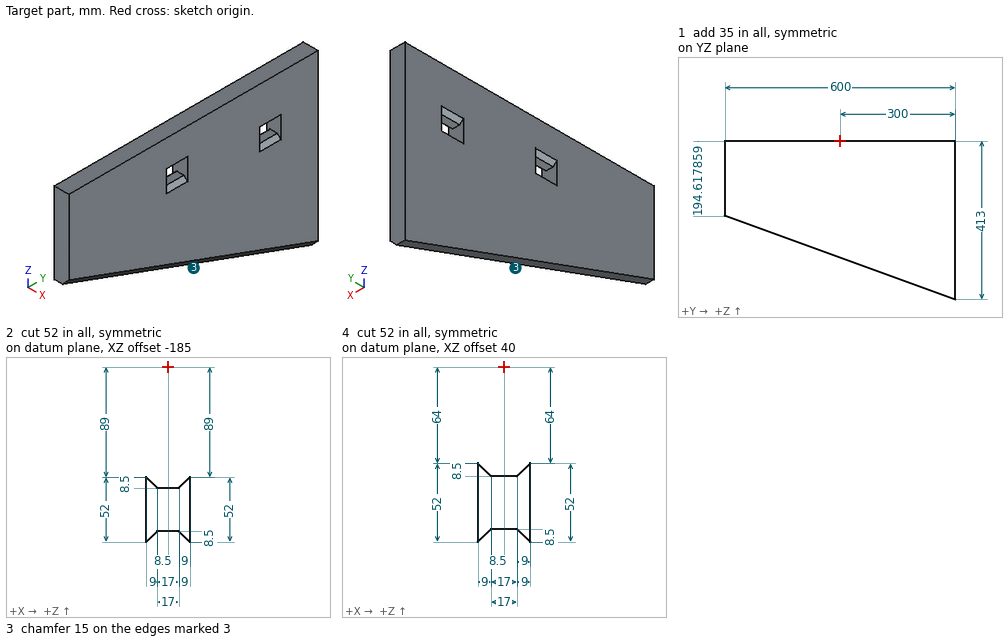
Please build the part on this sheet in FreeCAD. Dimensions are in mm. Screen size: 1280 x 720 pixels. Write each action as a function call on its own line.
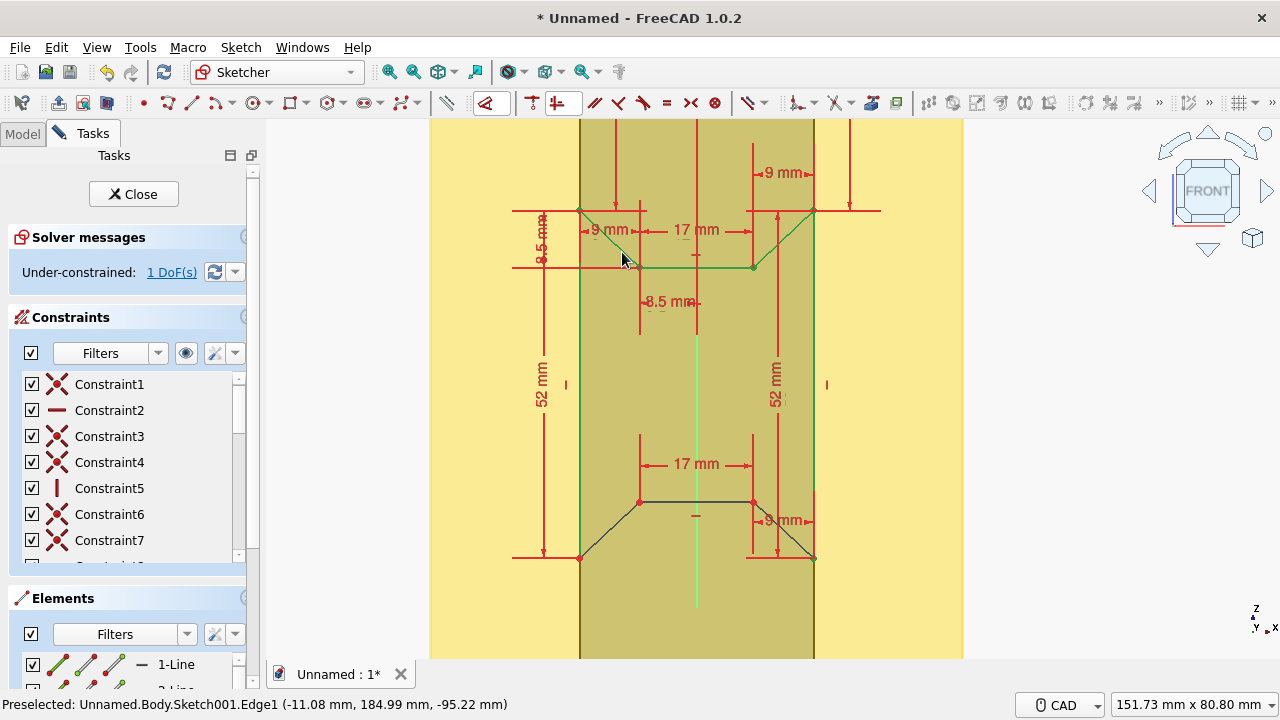
click(796, 541)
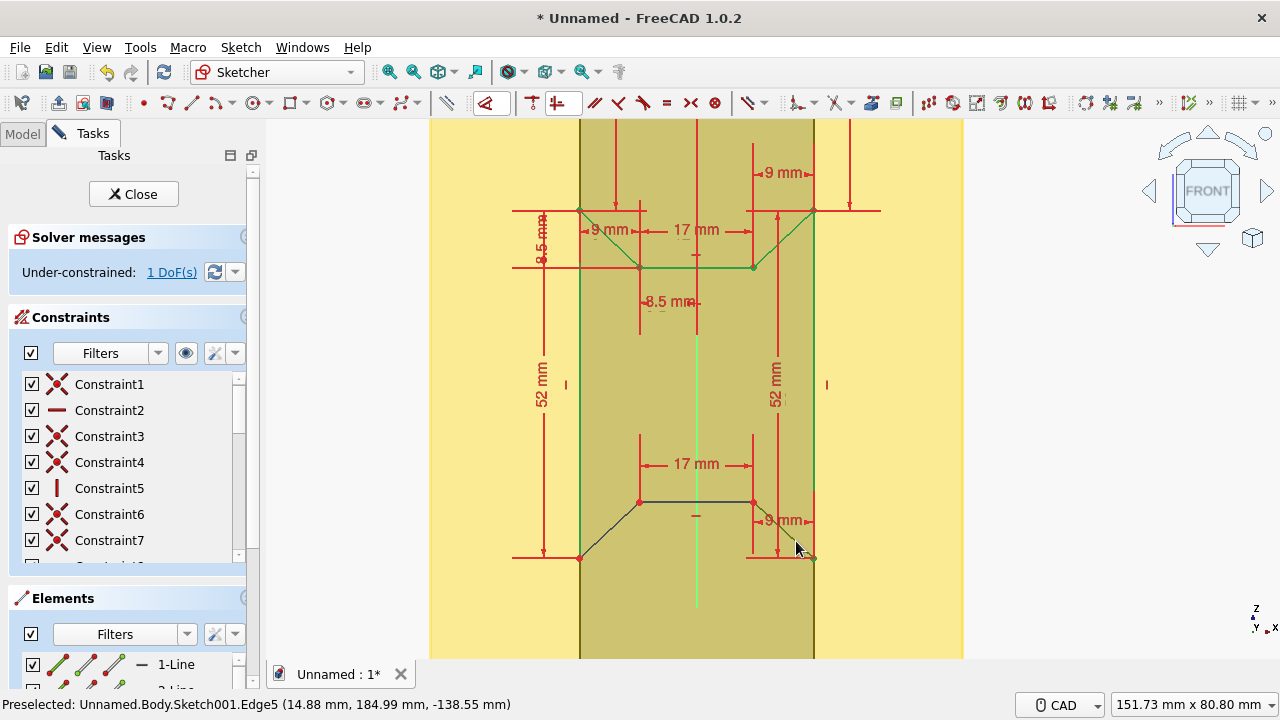
click(504, 104)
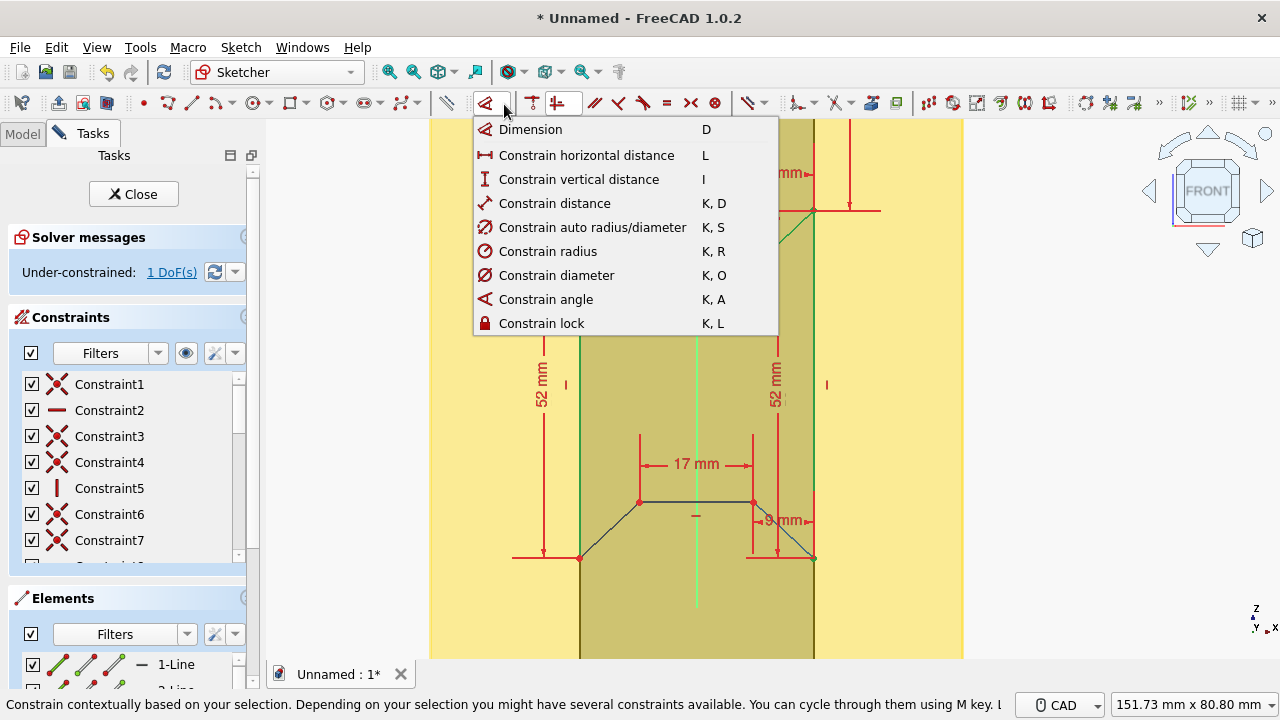
click(626, 179)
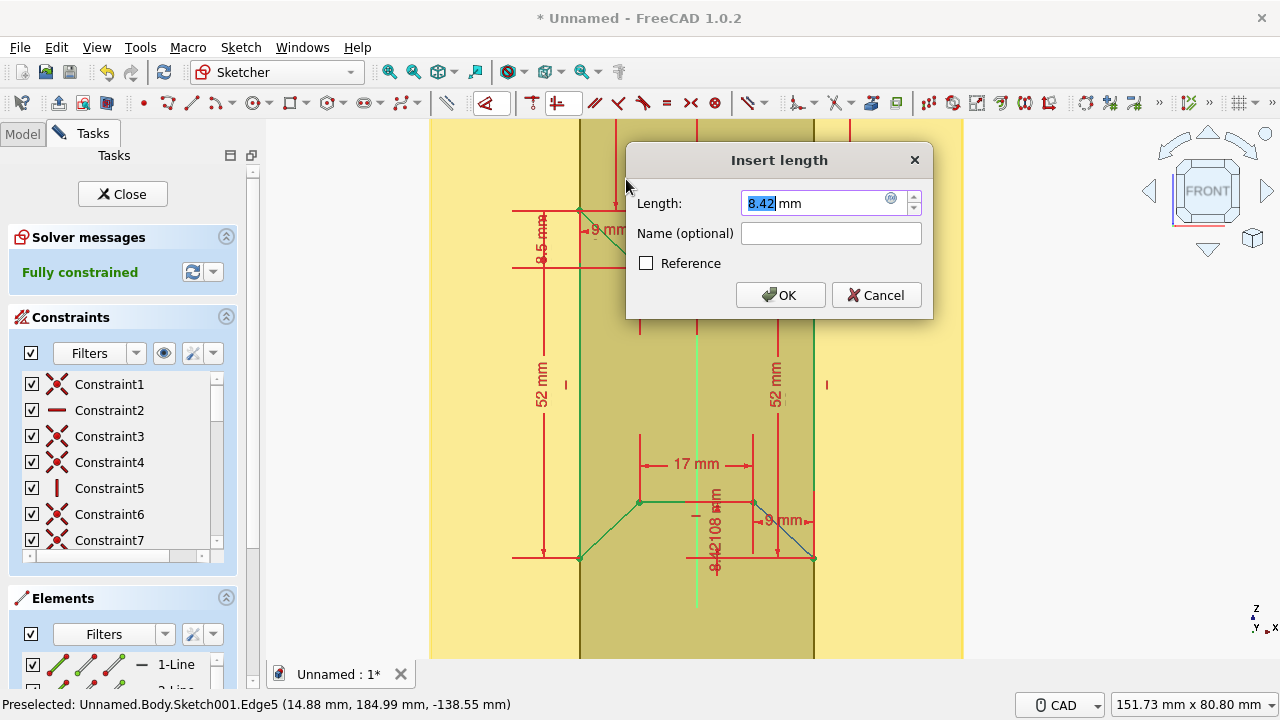
text(8.5)
key(Return)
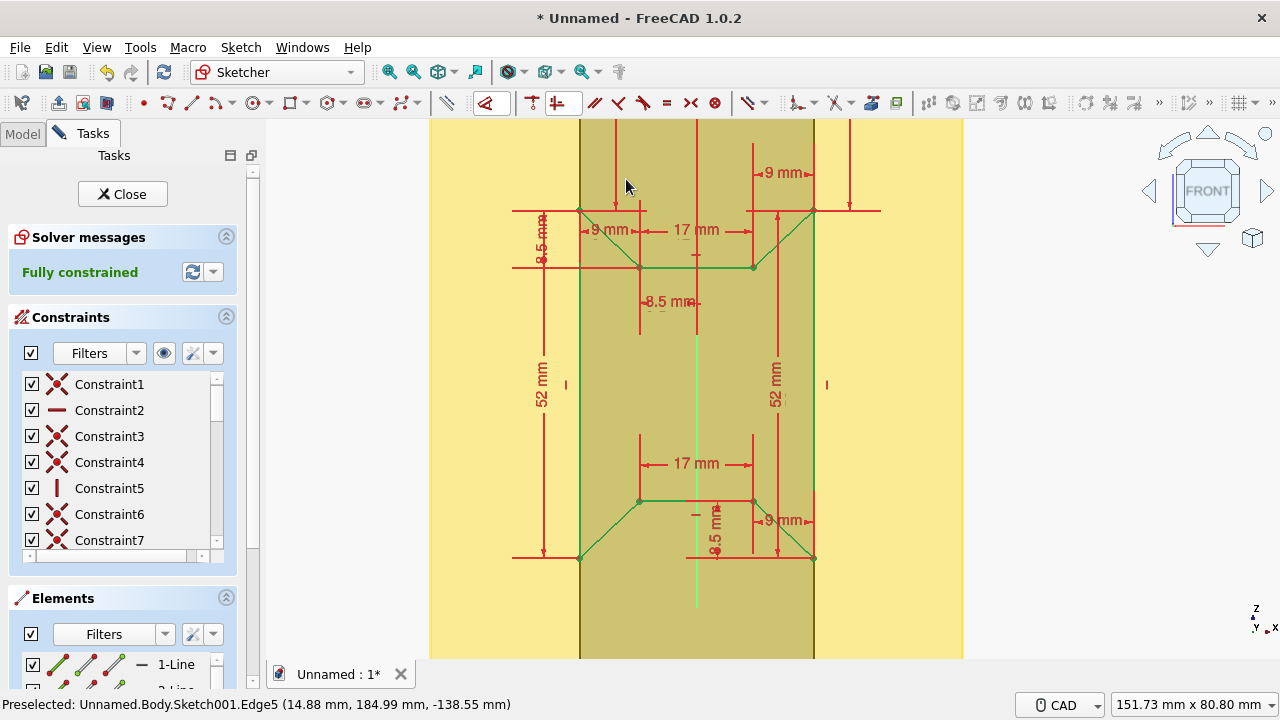
click(123, 194)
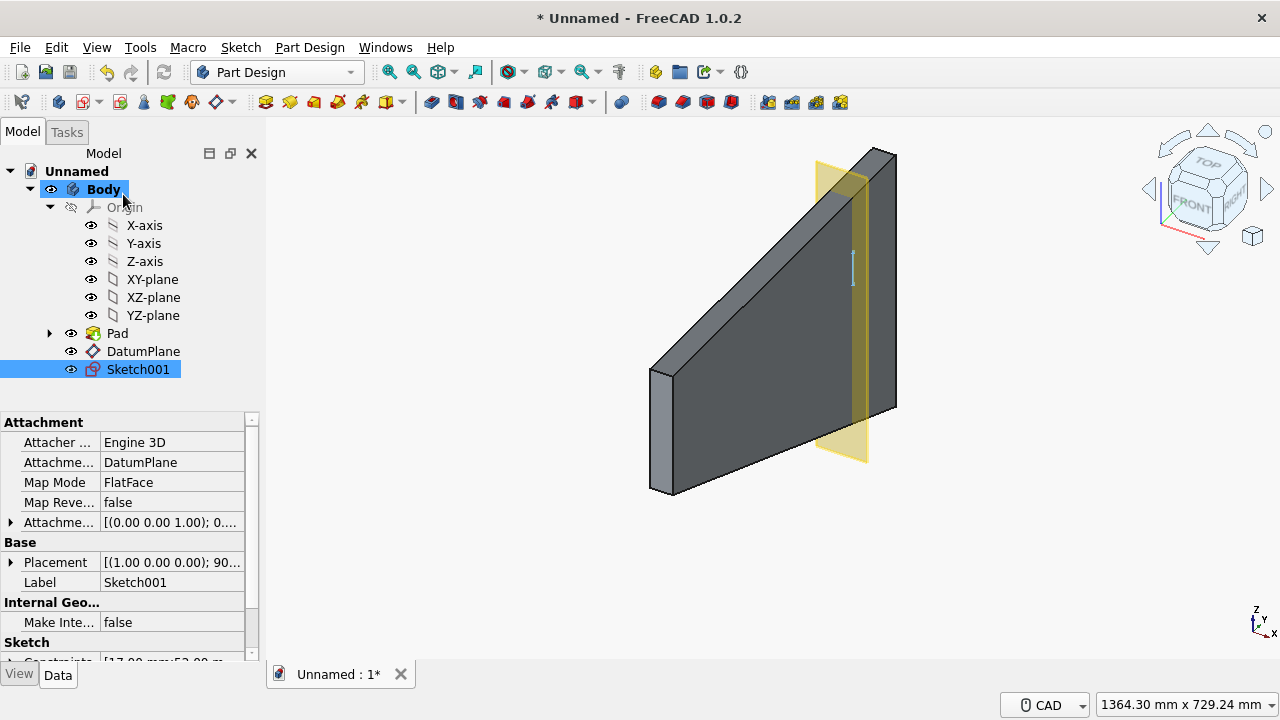
click(432, 102)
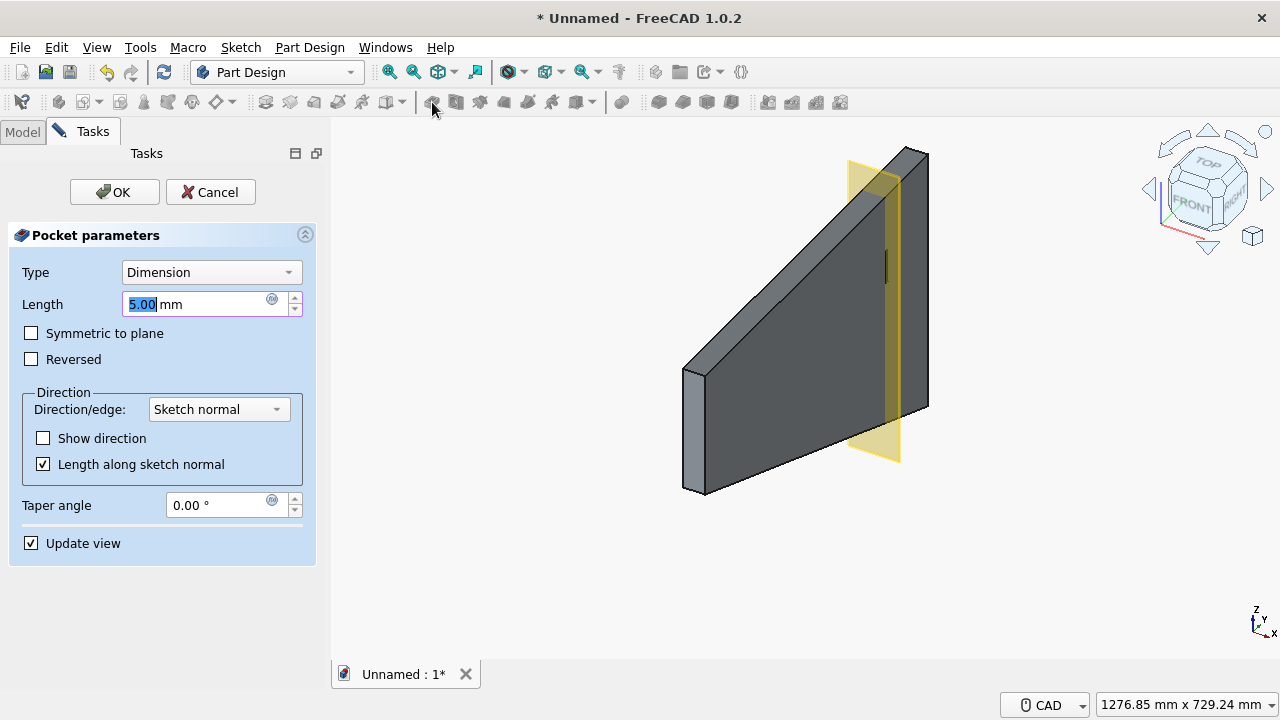
text(52)
key(Tab)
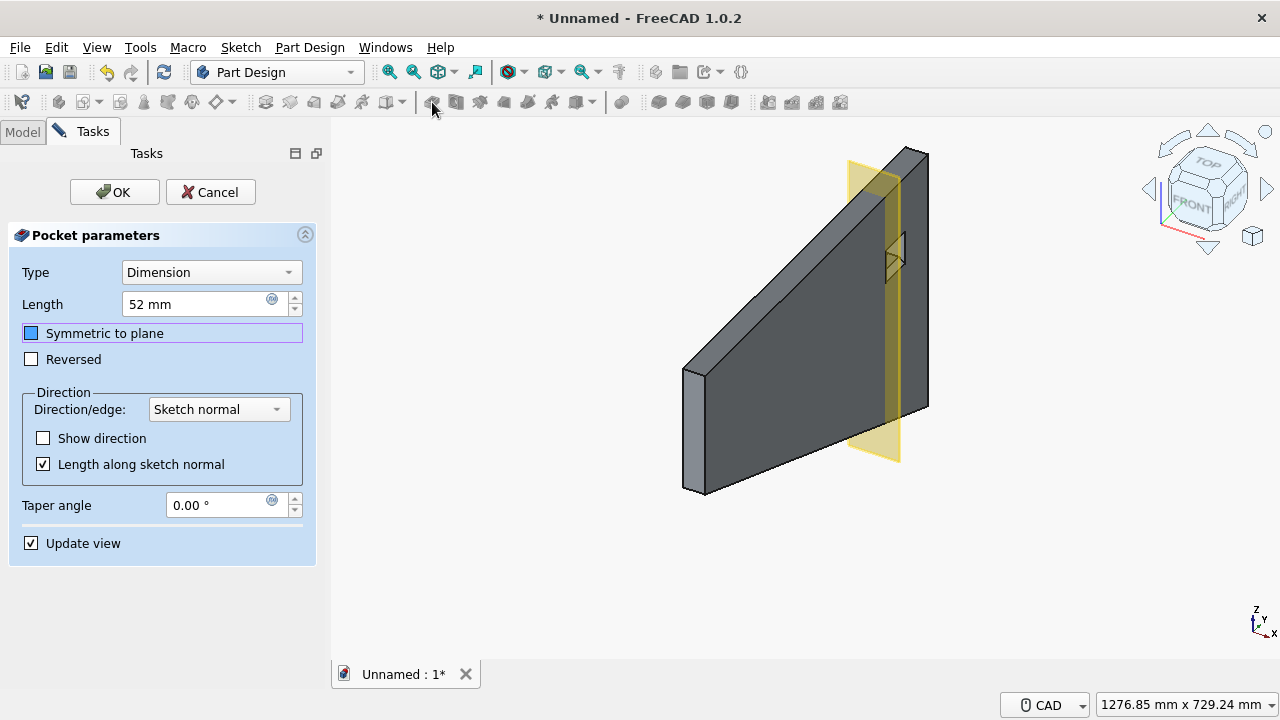
click(30, 333)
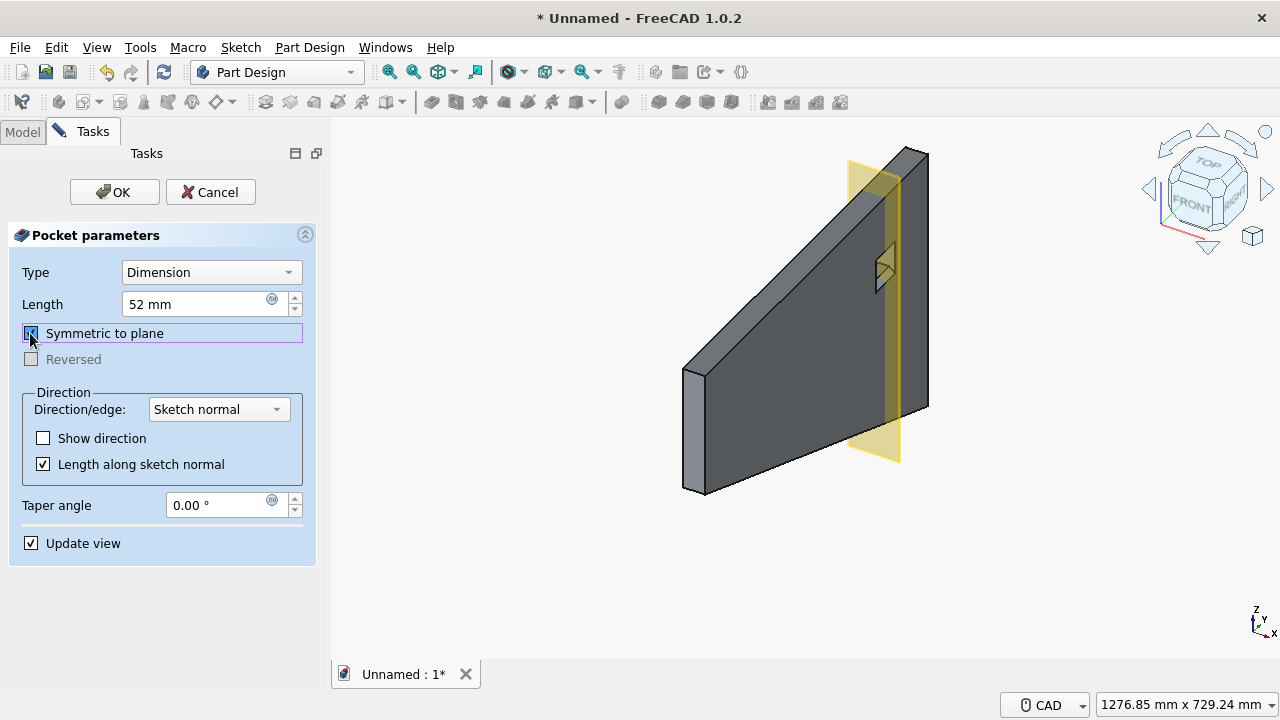
click(115, 192)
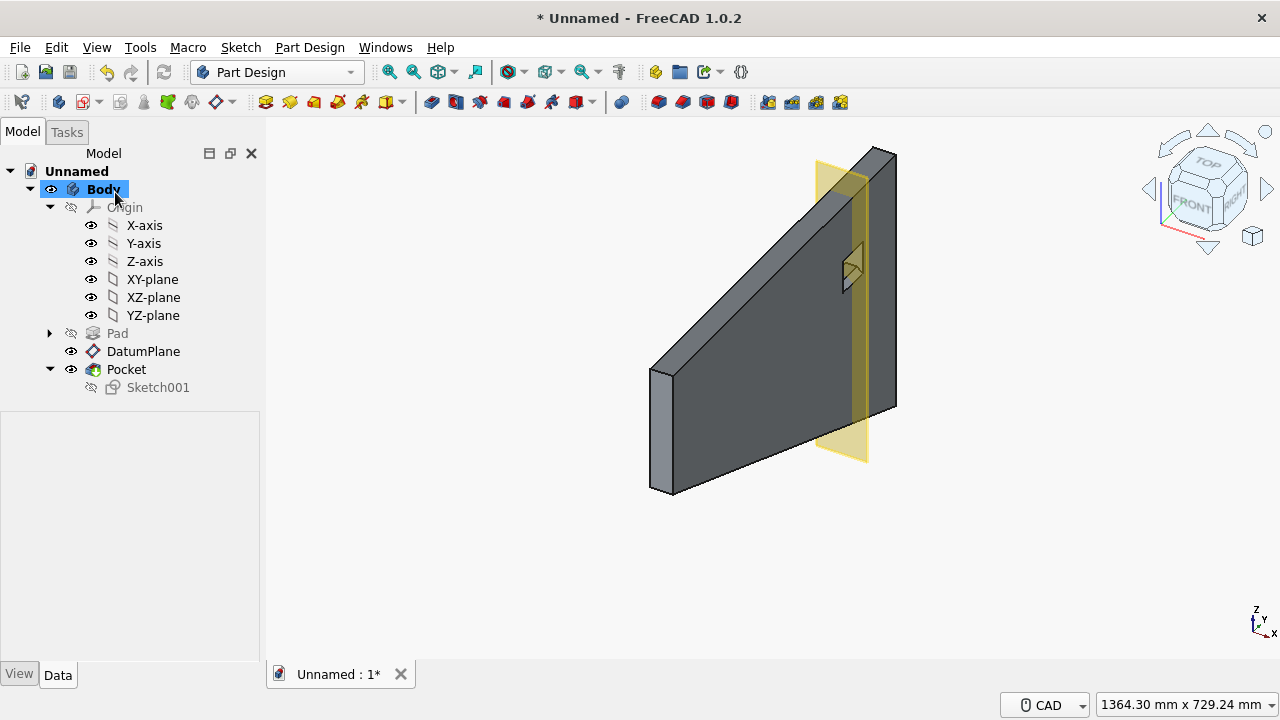
click(116, 351)
key(space)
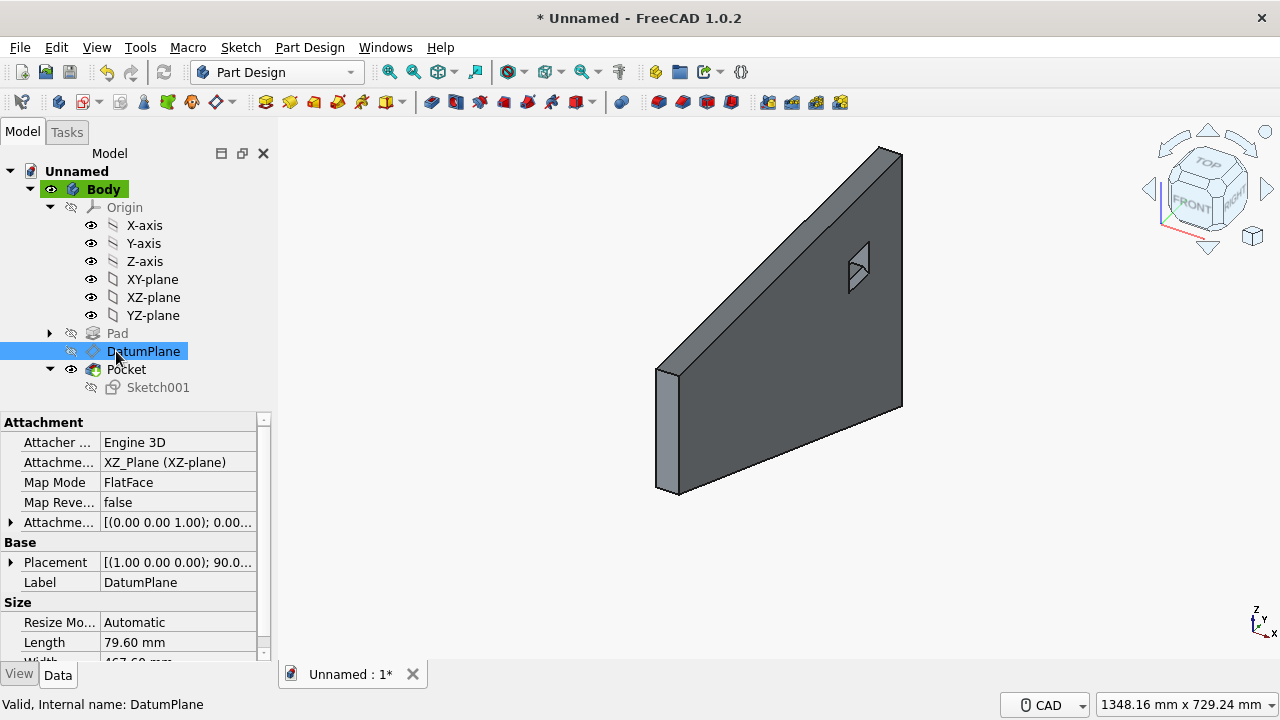
key(0)